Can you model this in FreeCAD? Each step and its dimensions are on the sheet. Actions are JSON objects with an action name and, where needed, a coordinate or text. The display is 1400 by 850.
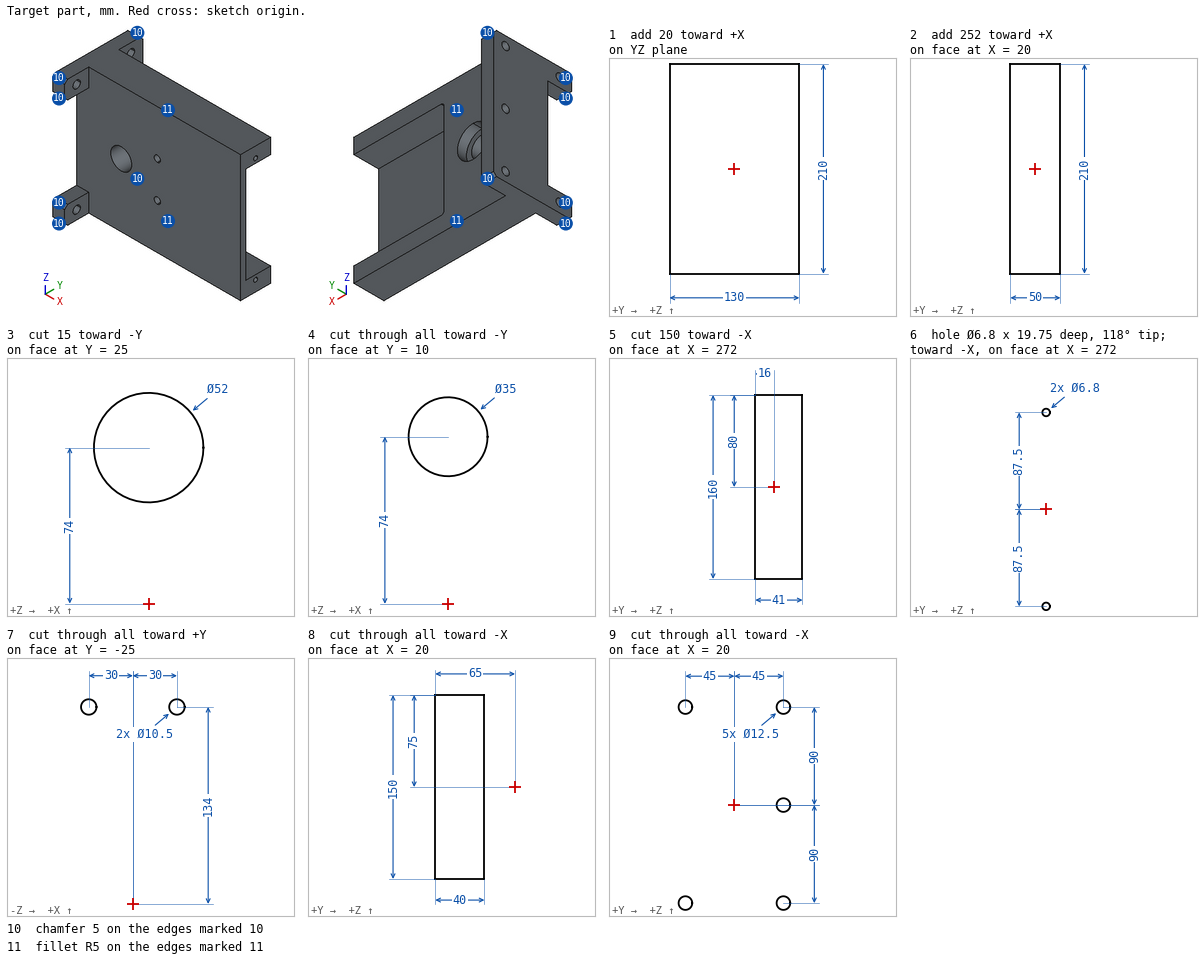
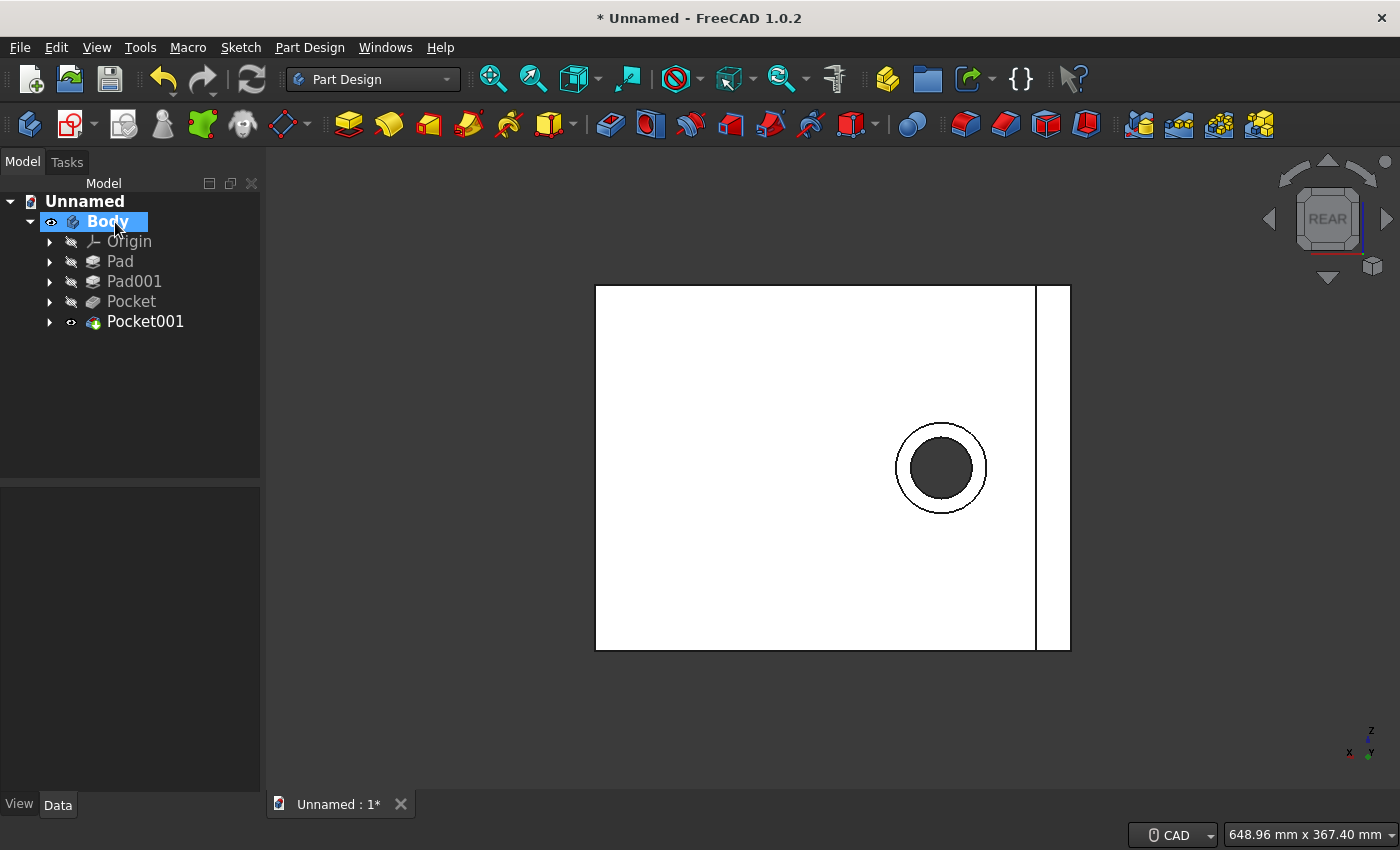
{"action": "key", "text": "0"}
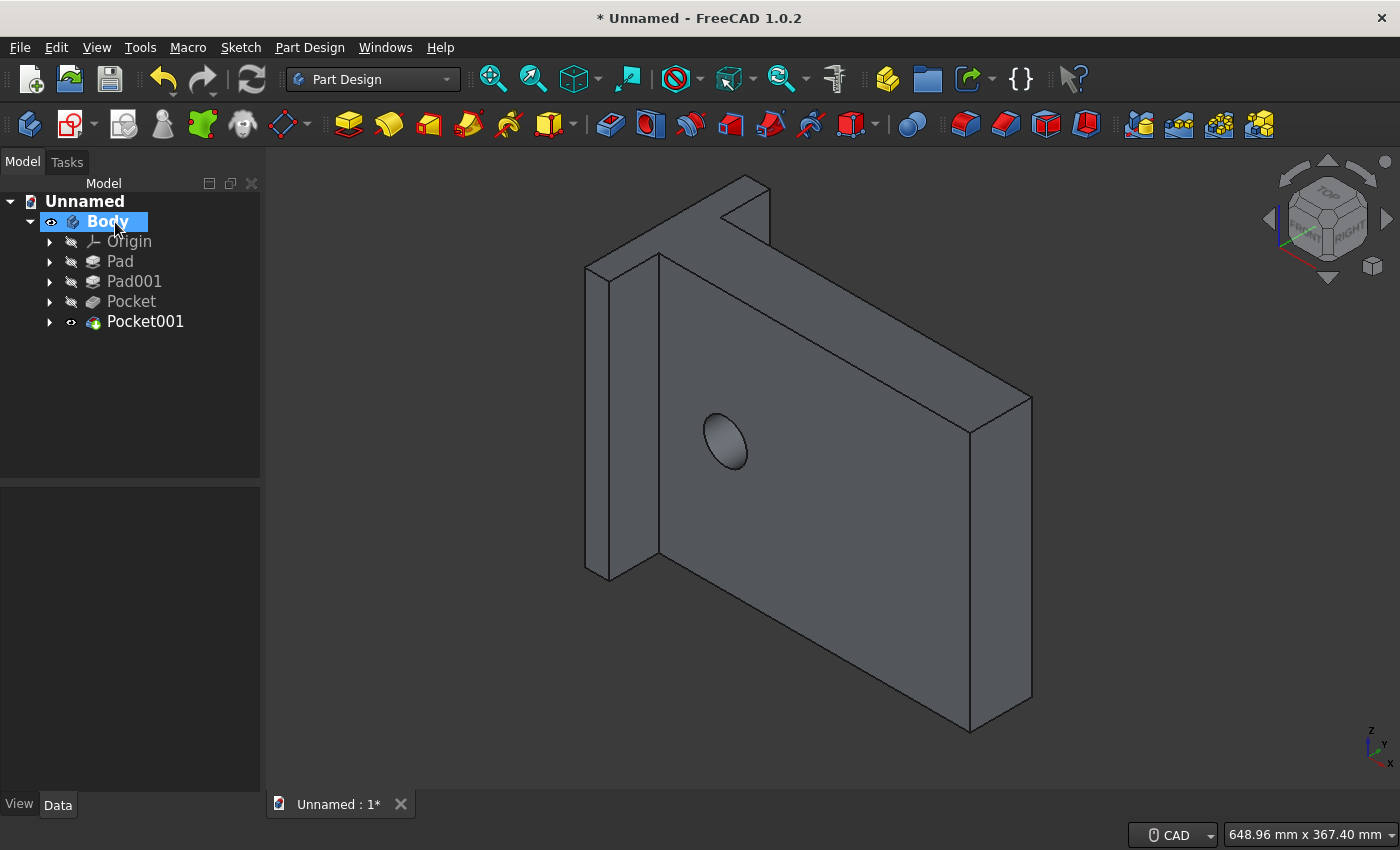
{"action": "left_click", "coordinate": [1001, 607]}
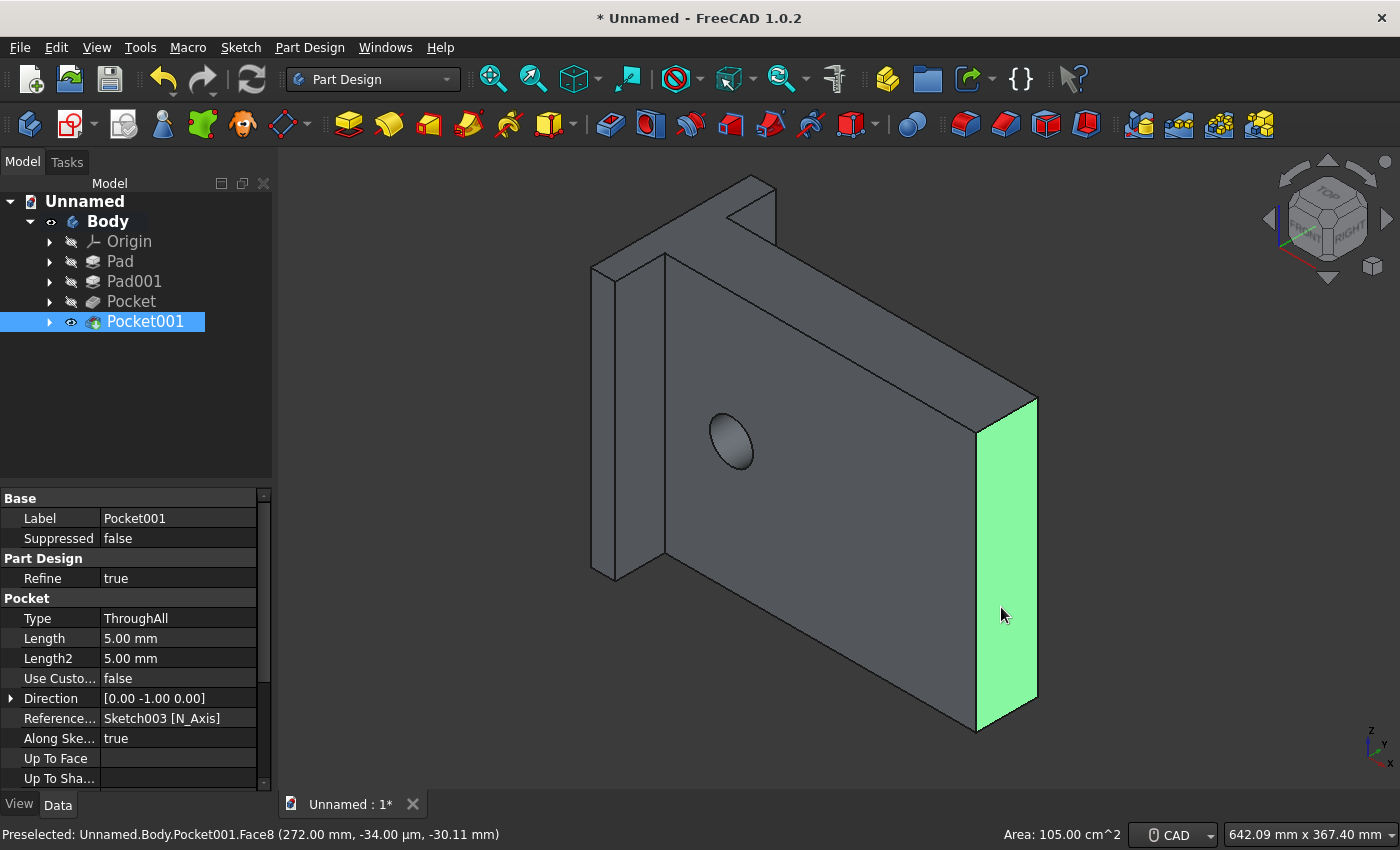
{"action": "left_click", "coordinate": [70, 124]}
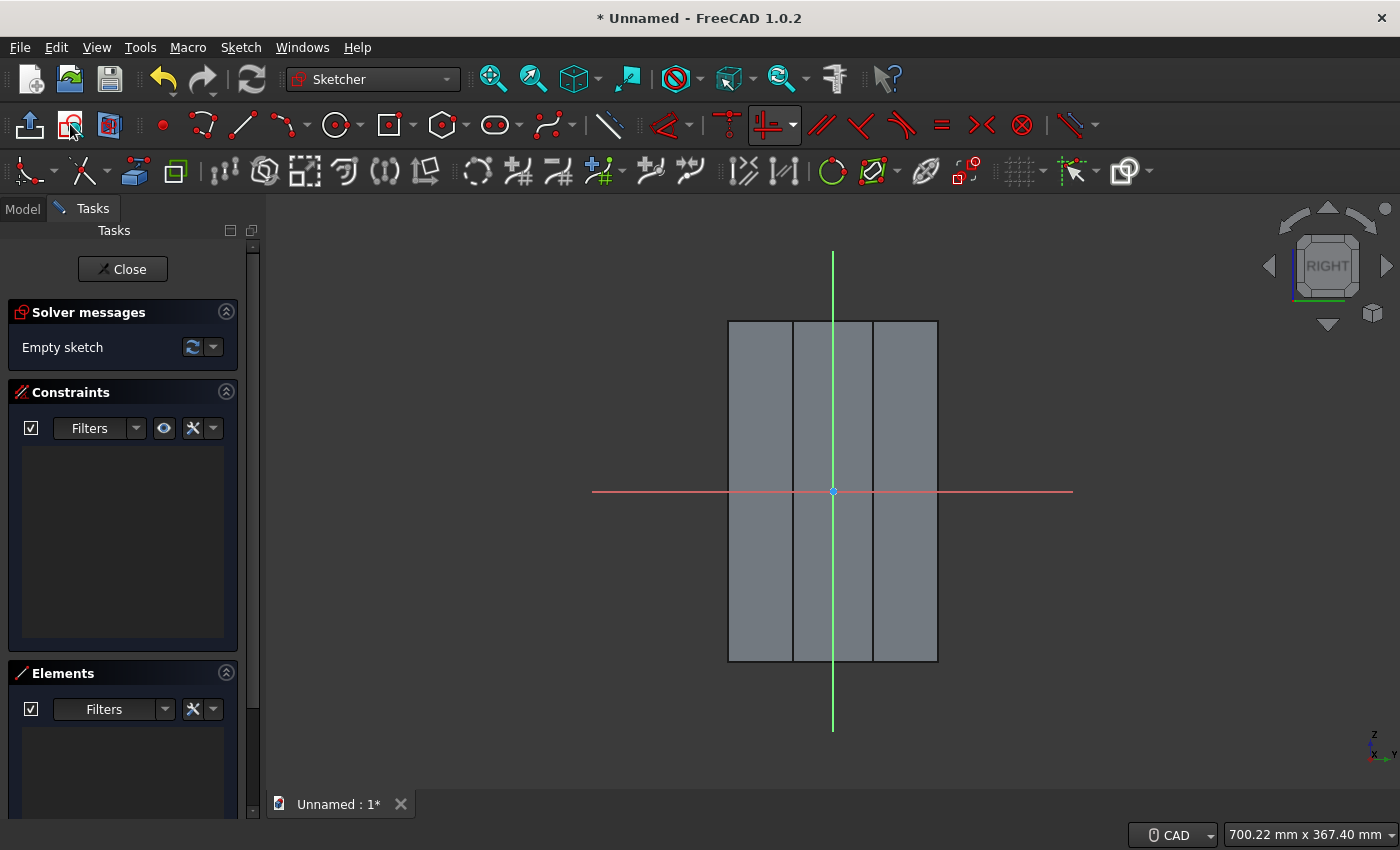
{"action": "scroll", "coordinate": [994, 492], "scroll_direction": "up", "scroll_amount": 2}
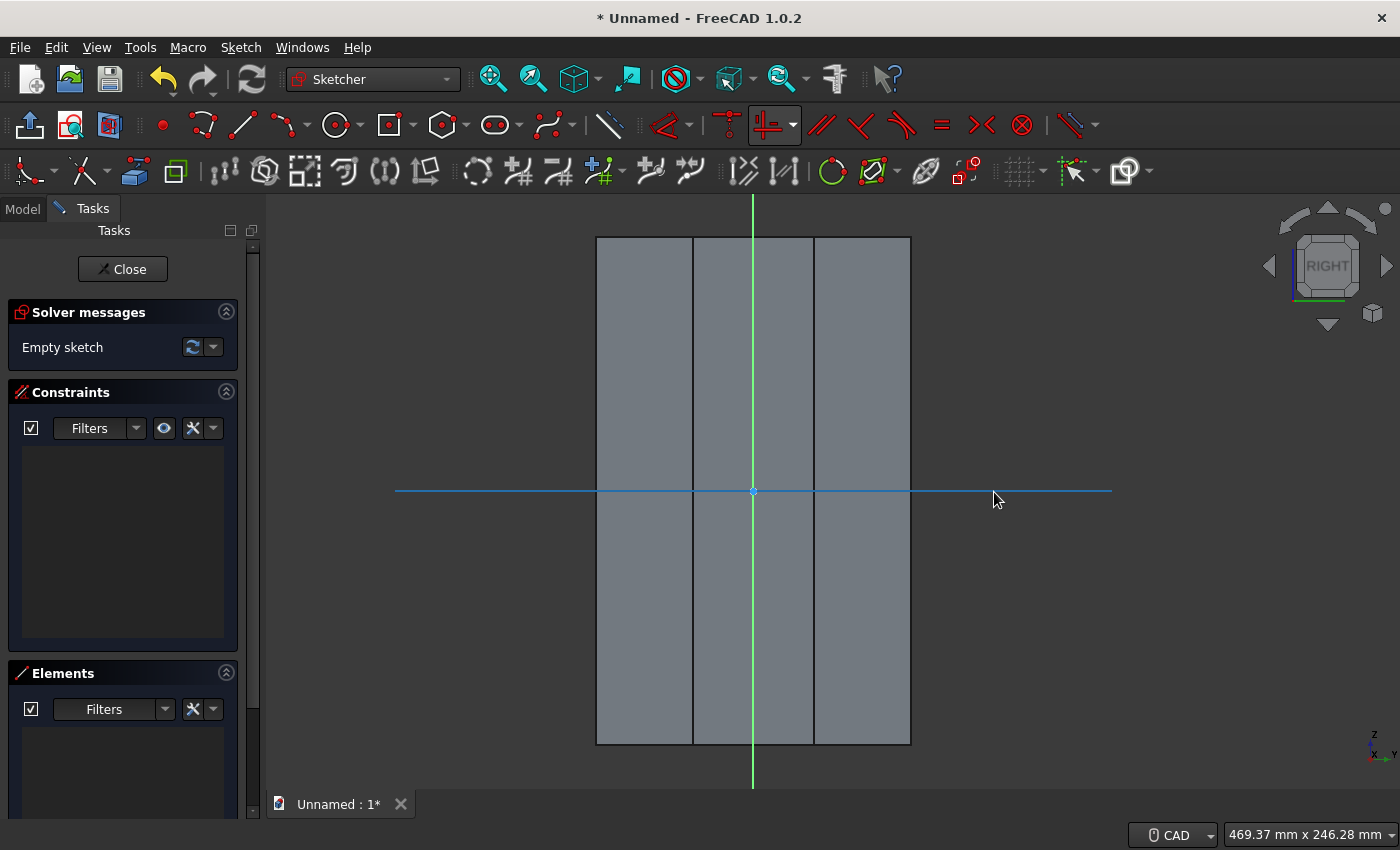
{"action": "key", "text": "g r"}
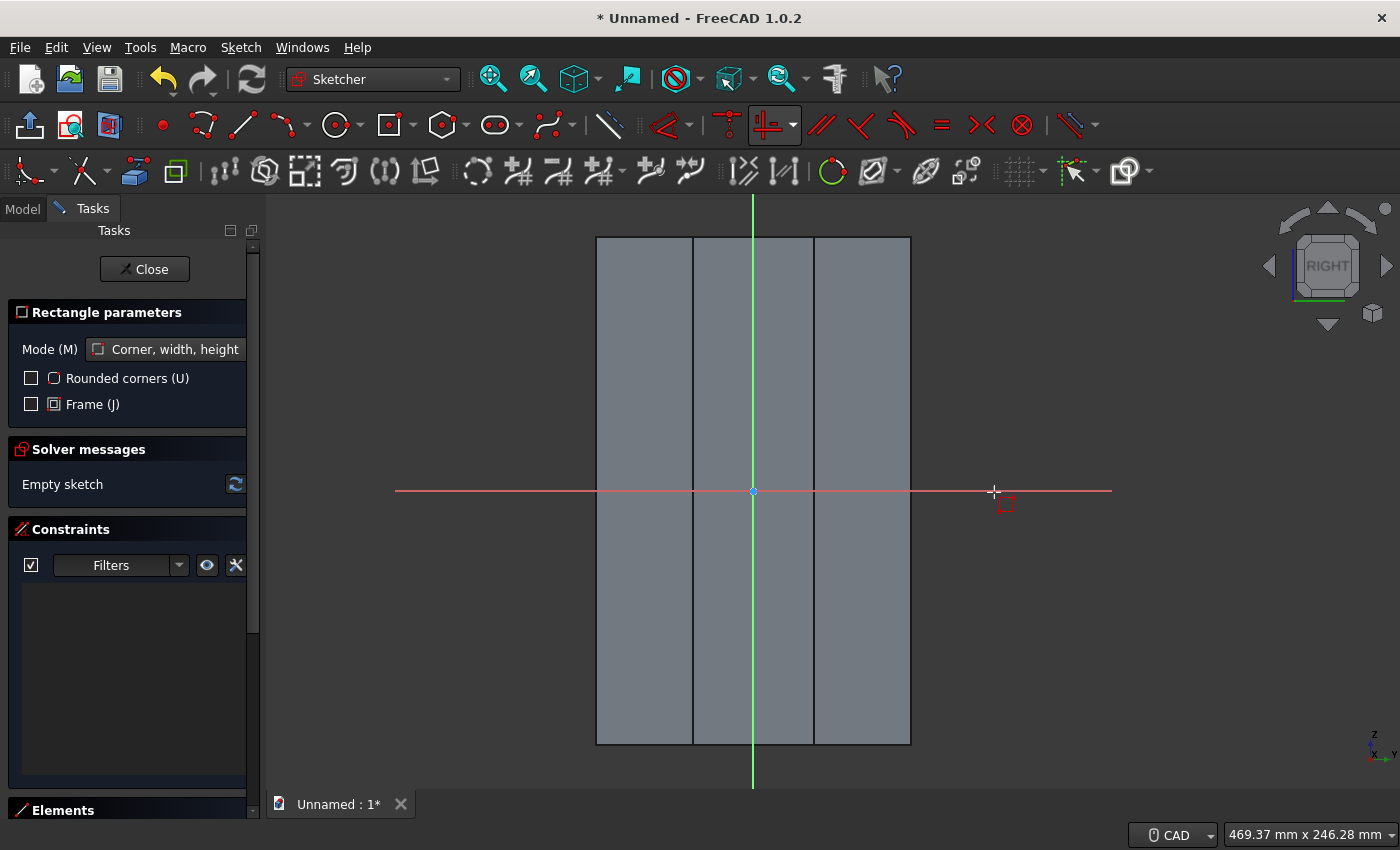
{"action": "left_click", "coordinate": [715, 298]}
{"action": "left_click", "coordinate": [814, 684]}
{"action": "key", "text": "Escape"}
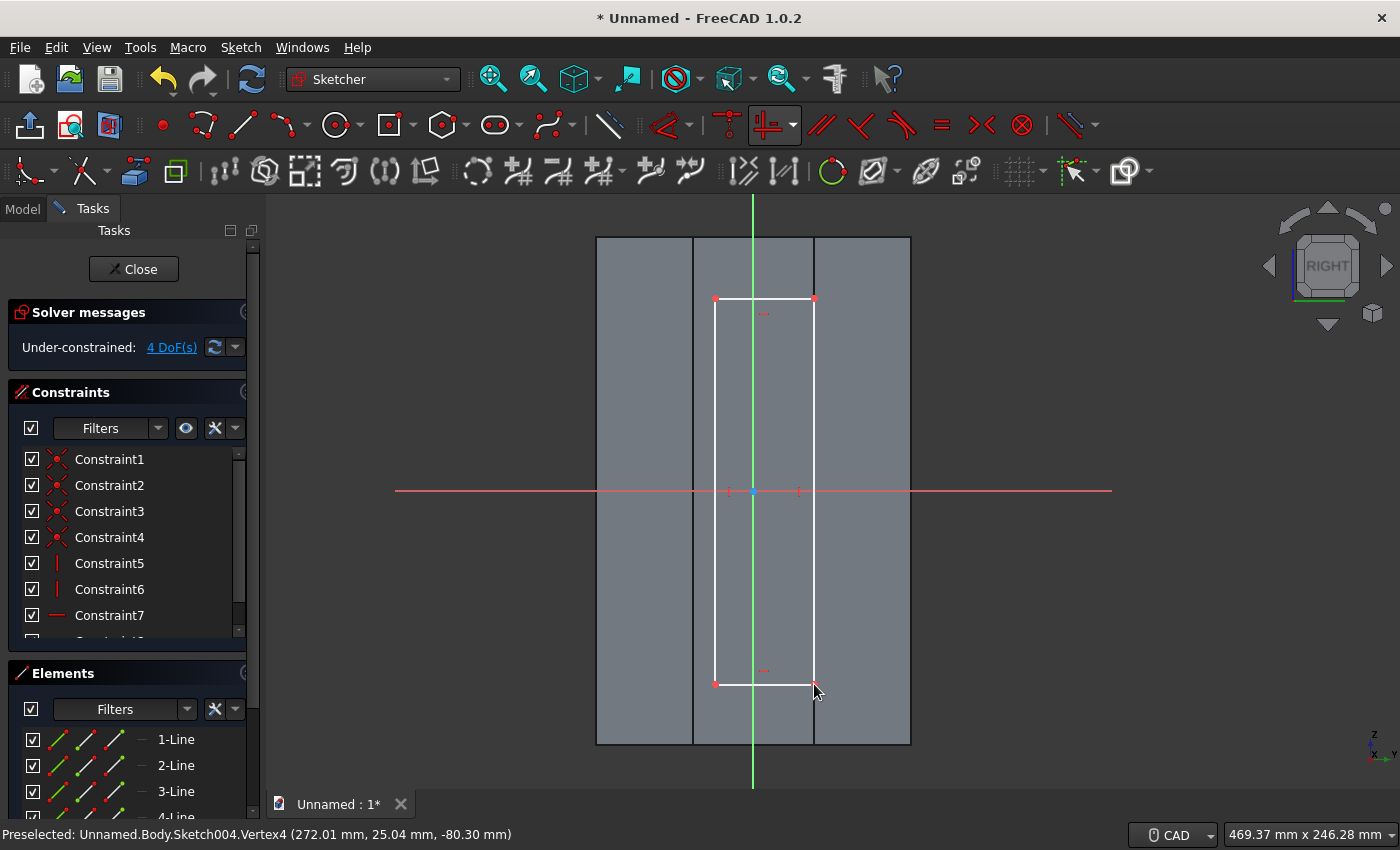
{"action": "left_click", "coordinate": [664, 126]}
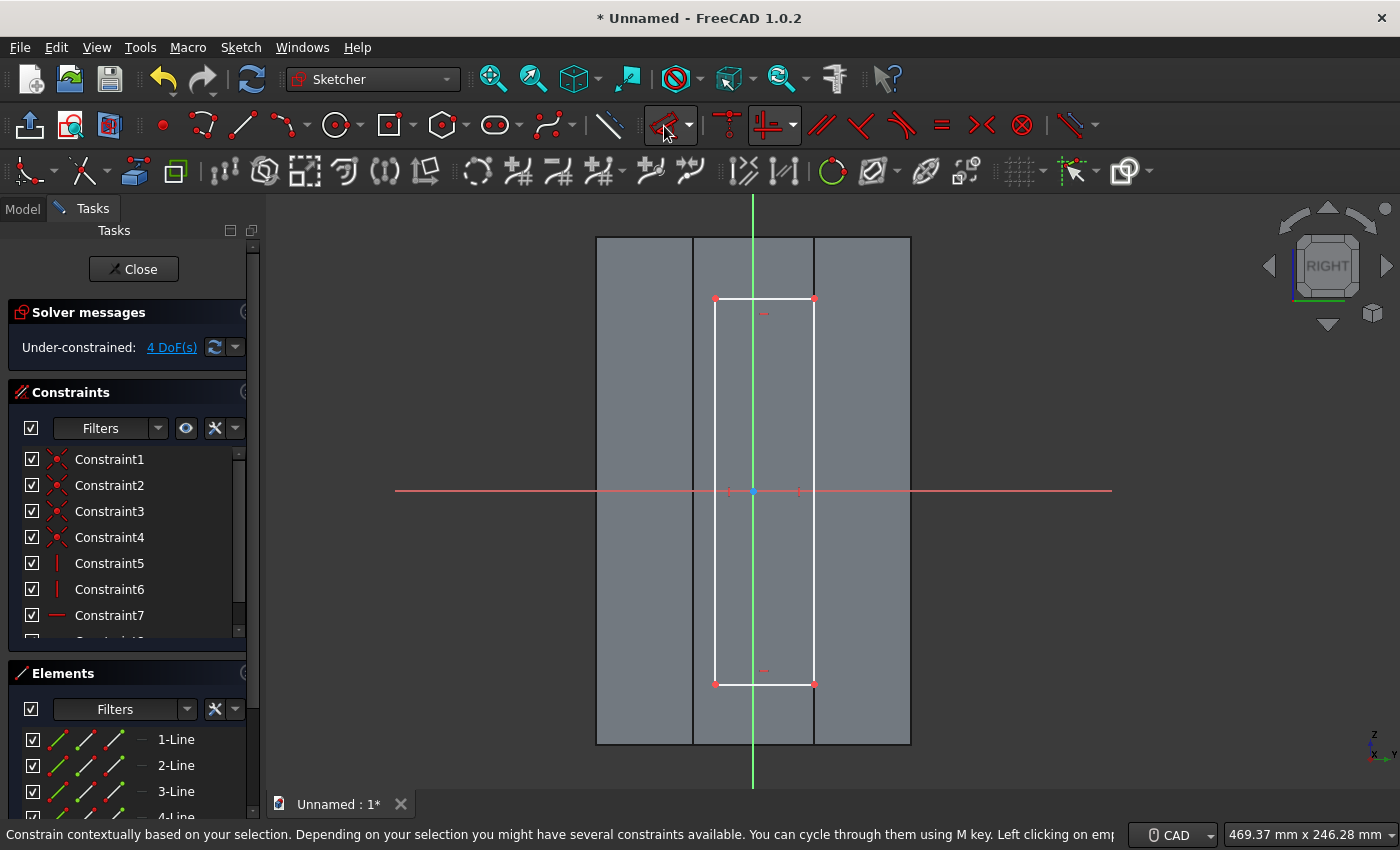
{"action": "left_click", "coordinate": [784, 685]}
{"action": "left_click", "coordinate": [787, 719]}